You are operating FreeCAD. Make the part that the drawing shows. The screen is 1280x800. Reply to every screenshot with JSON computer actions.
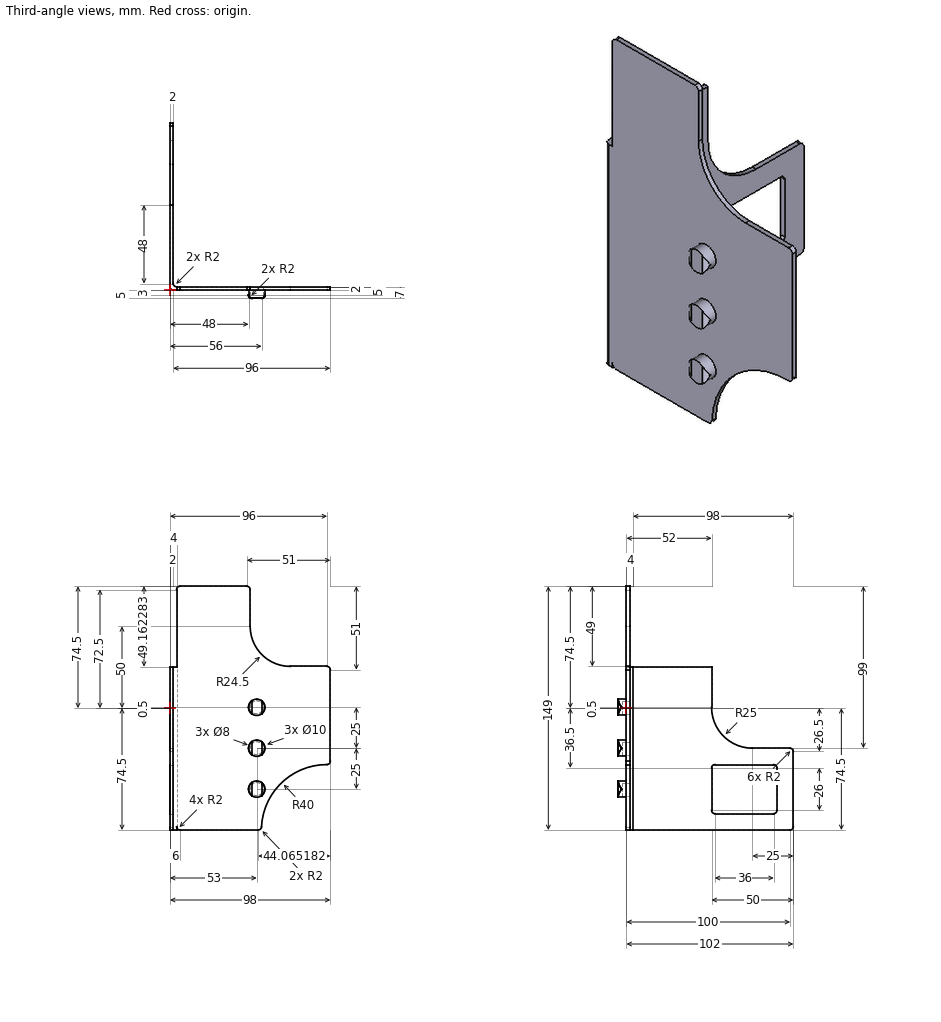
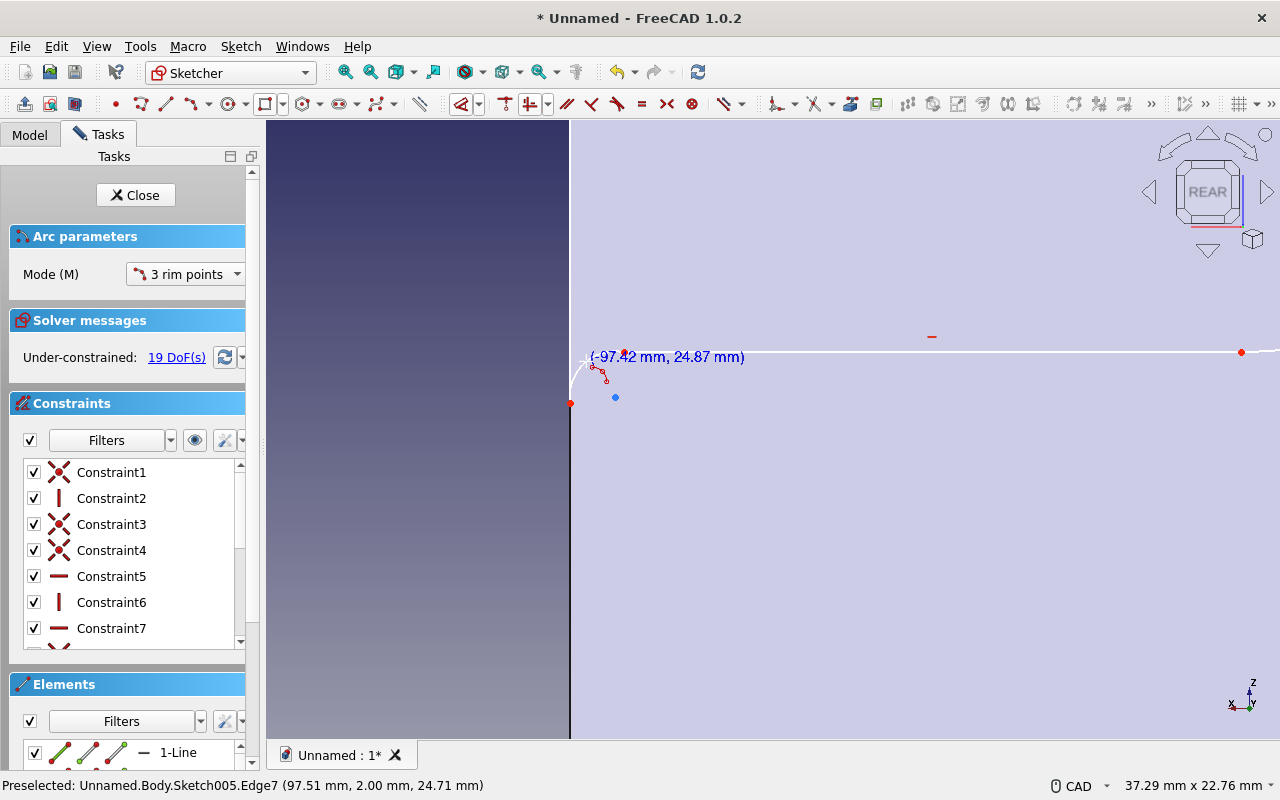
{"action": "left_click", "coordinate": [141, 104]}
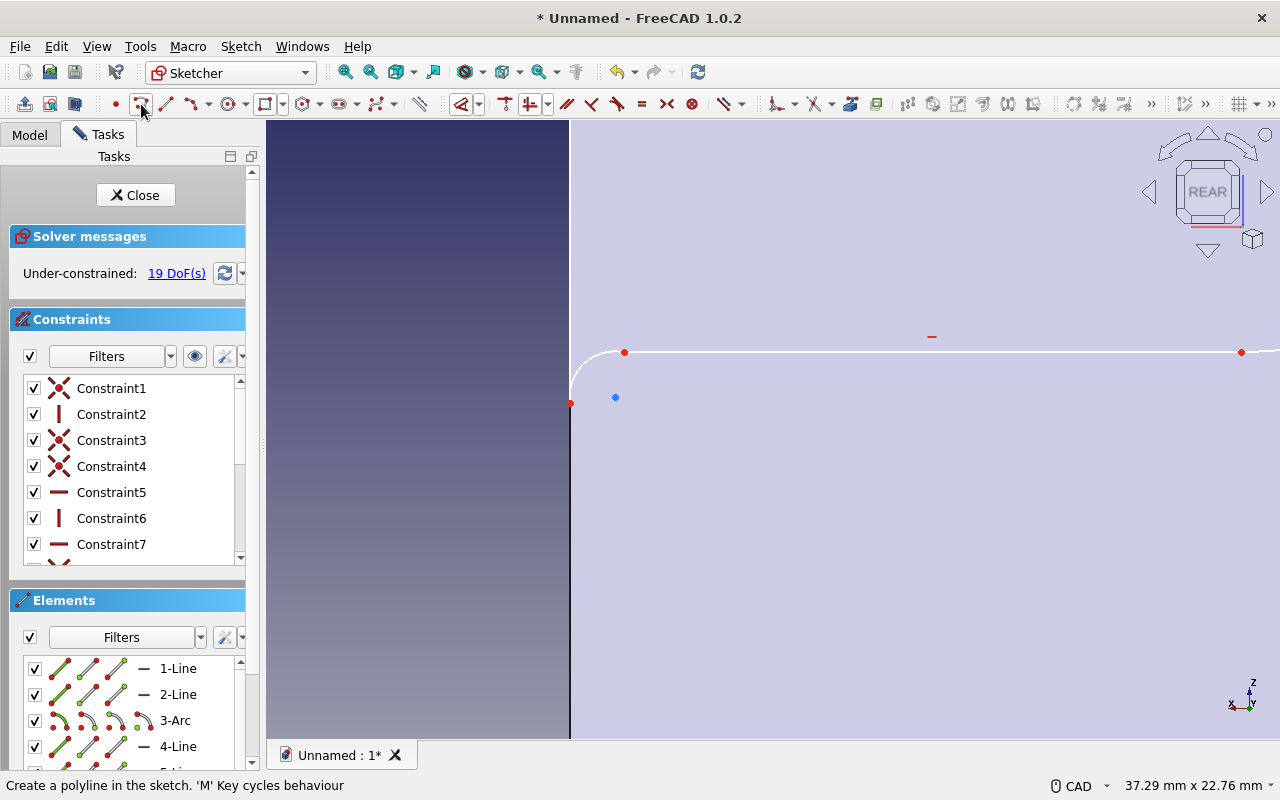
{"action": "scroll", "coordinate": [585, 369], "scroll_direction": "down", "scroll_amount": 12}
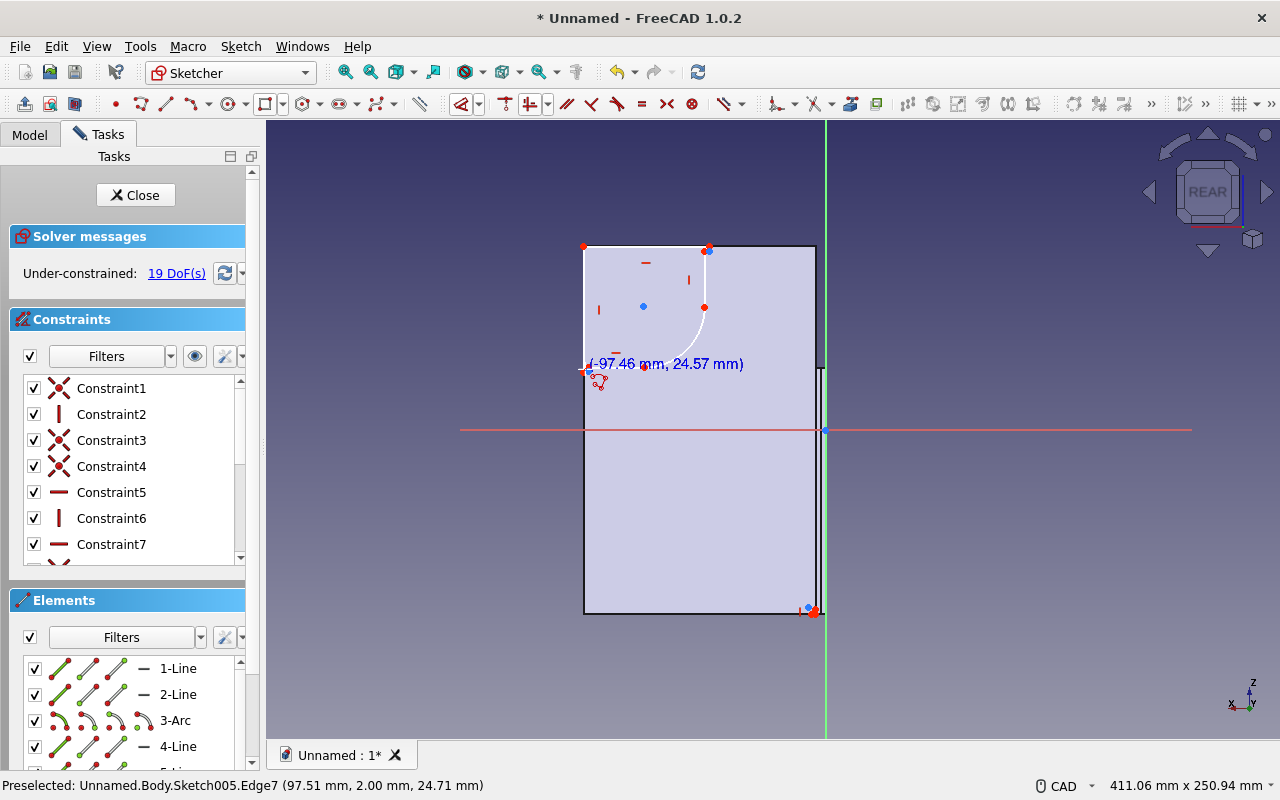
{"action": "scroll", "coordinate": [816, 251], "scroll_direction": "up", "scroll_amount": 3}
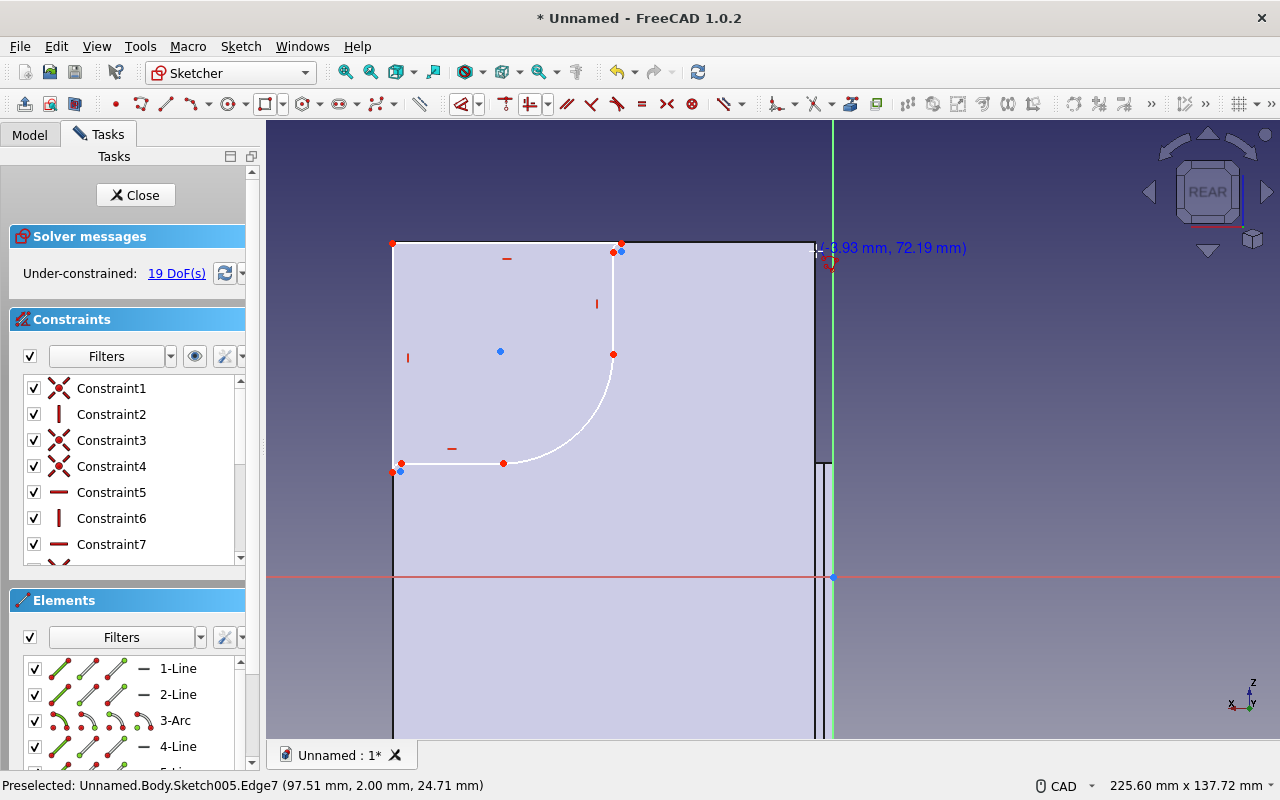
{"action": "left_click", "coordinate": [815, 251]}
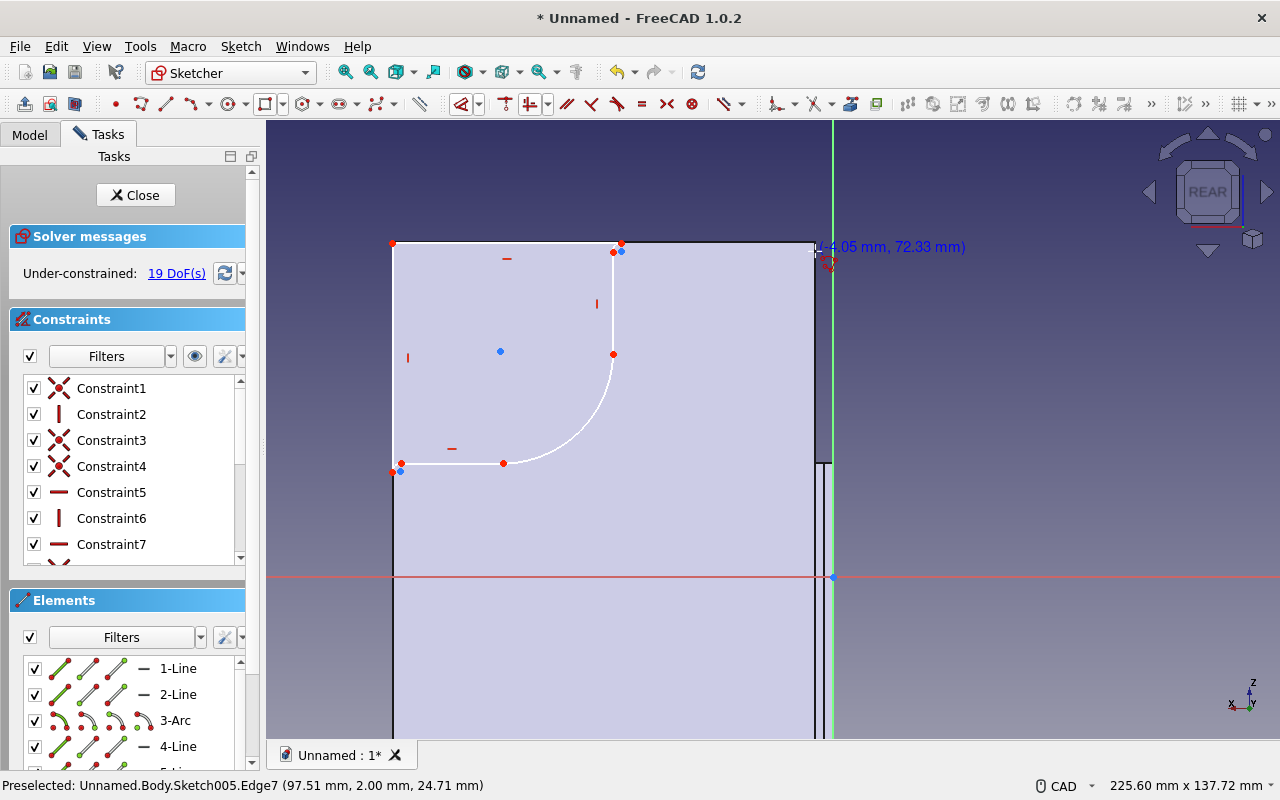
{"action": "scroll", "coordinate": [815, 242], "scroll_direction": "up", "scroll_amount": 3}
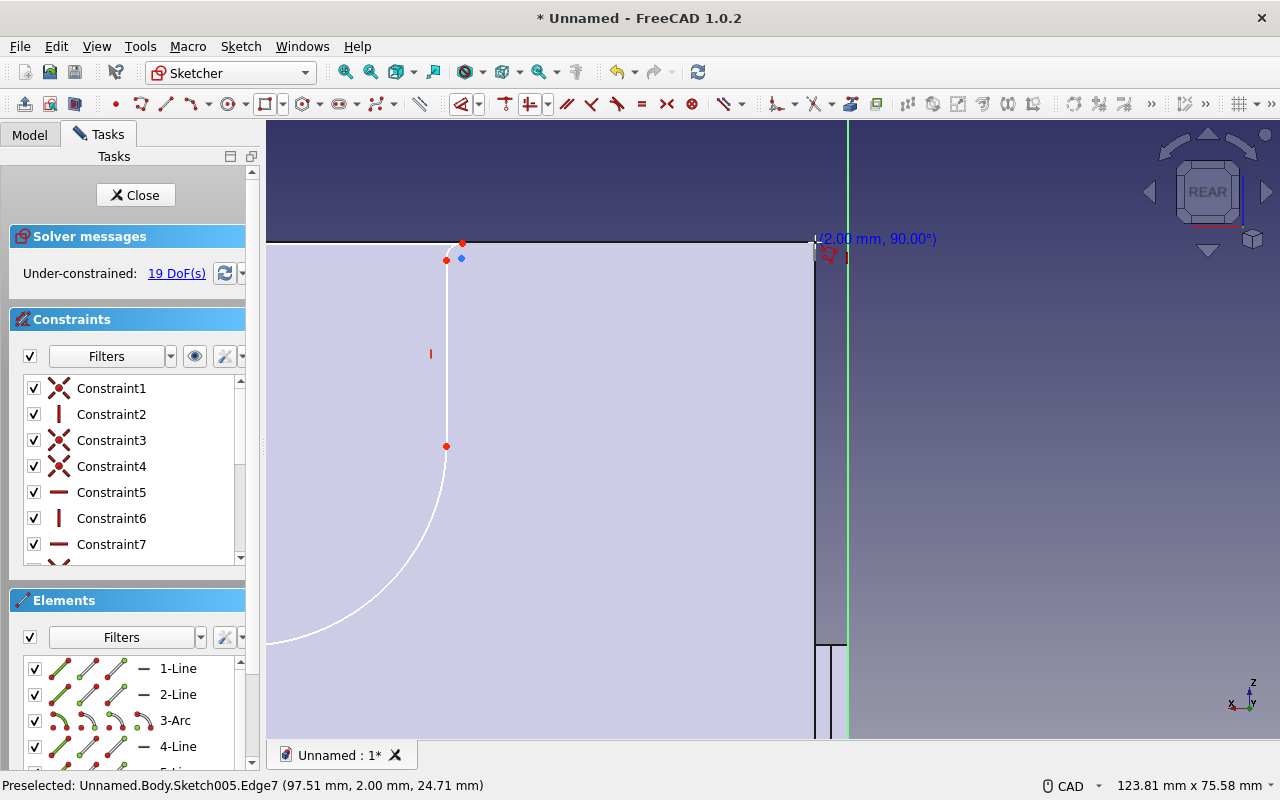
{"action": "left_click", "coordinate": [815, 242]}
{"action": "left_click", "coordinate": [799, 242]}
{"action": "right_click", "coordinate": [799, 242]}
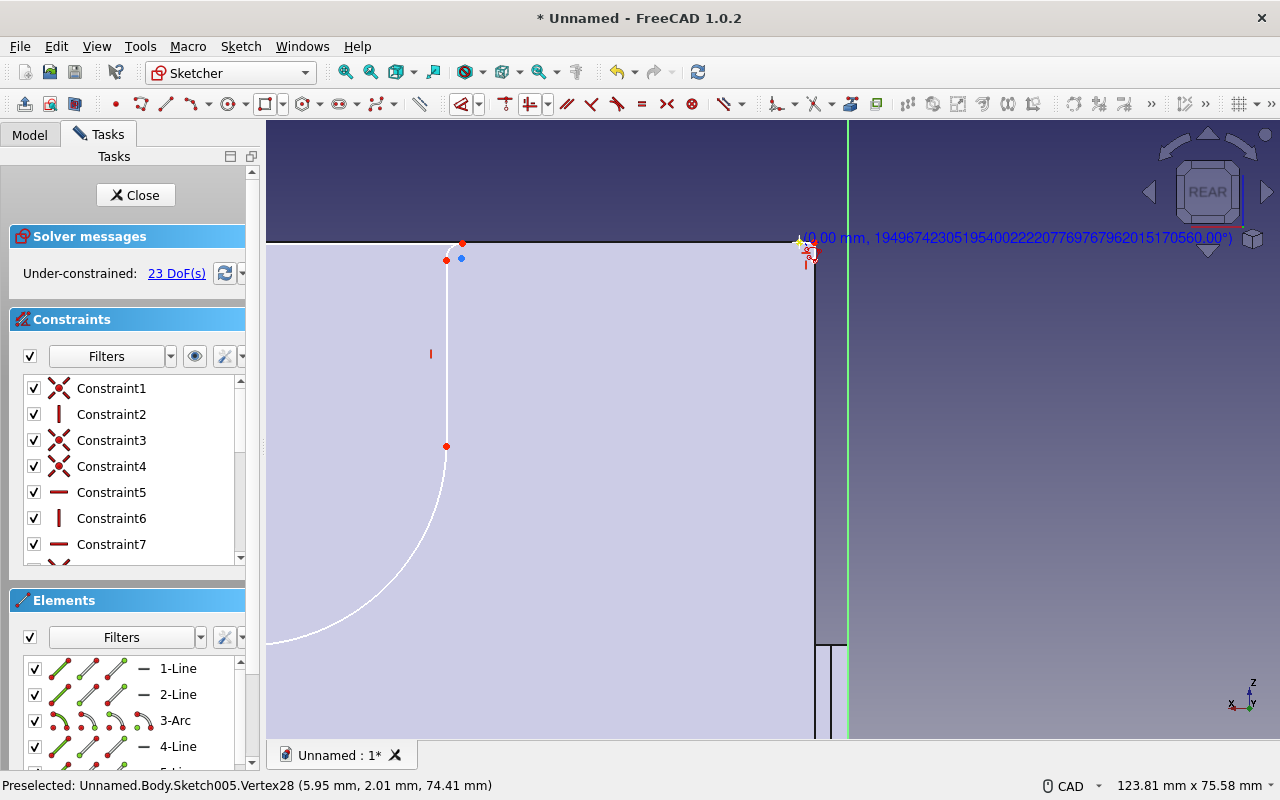
{"action": "key", "text": "g 3 a"}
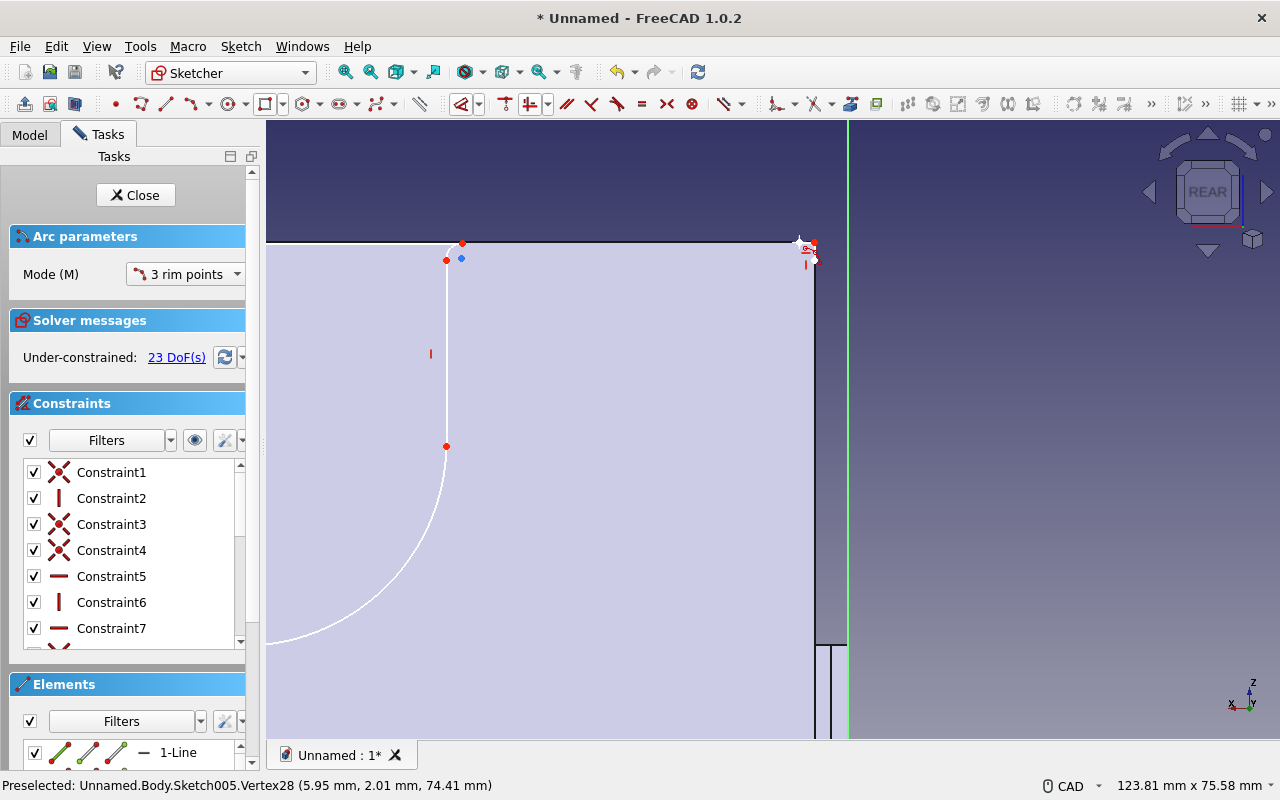
{"action": "scroll", "coordinate": [799, 242], "scroll_direction": "up", "scroll_amount": 4}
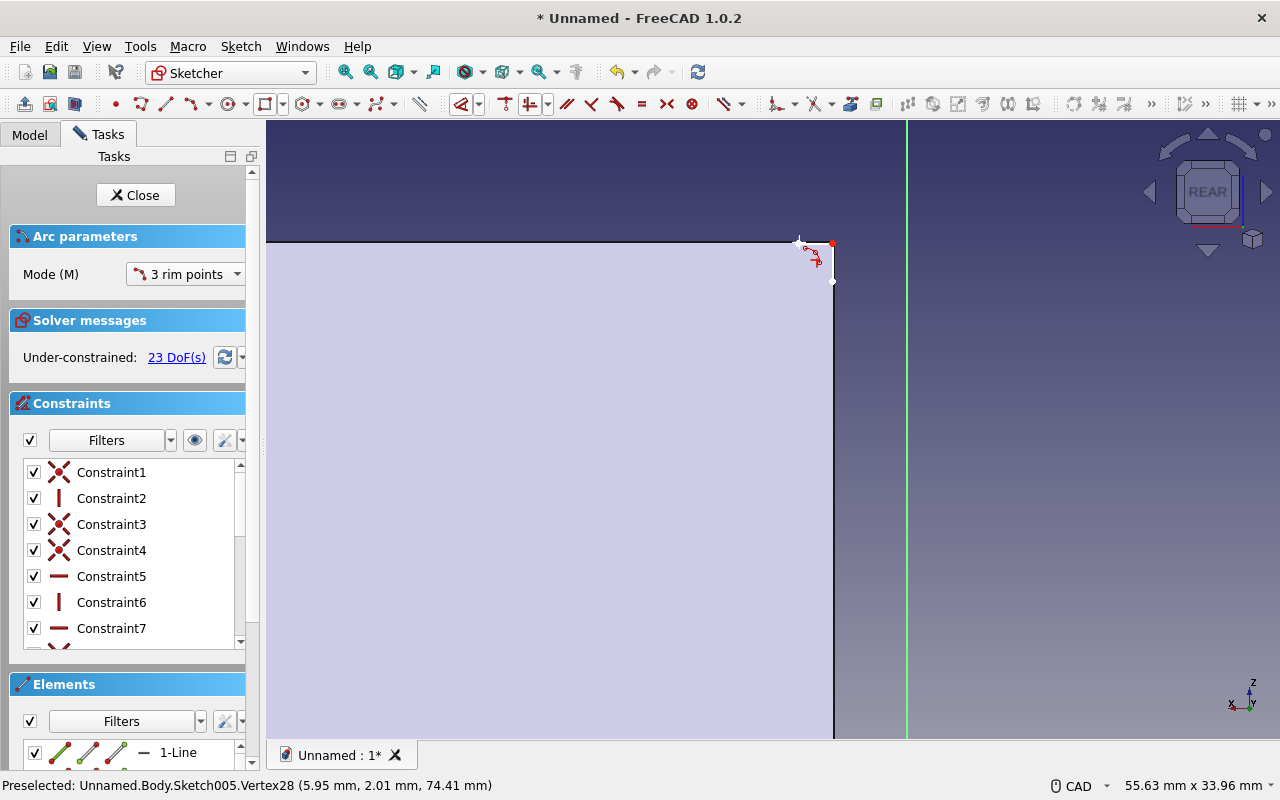
{"action": "left_click", "coordinate": [798, 244]}
{"action": "left_click", "coordinate": [833, 282]}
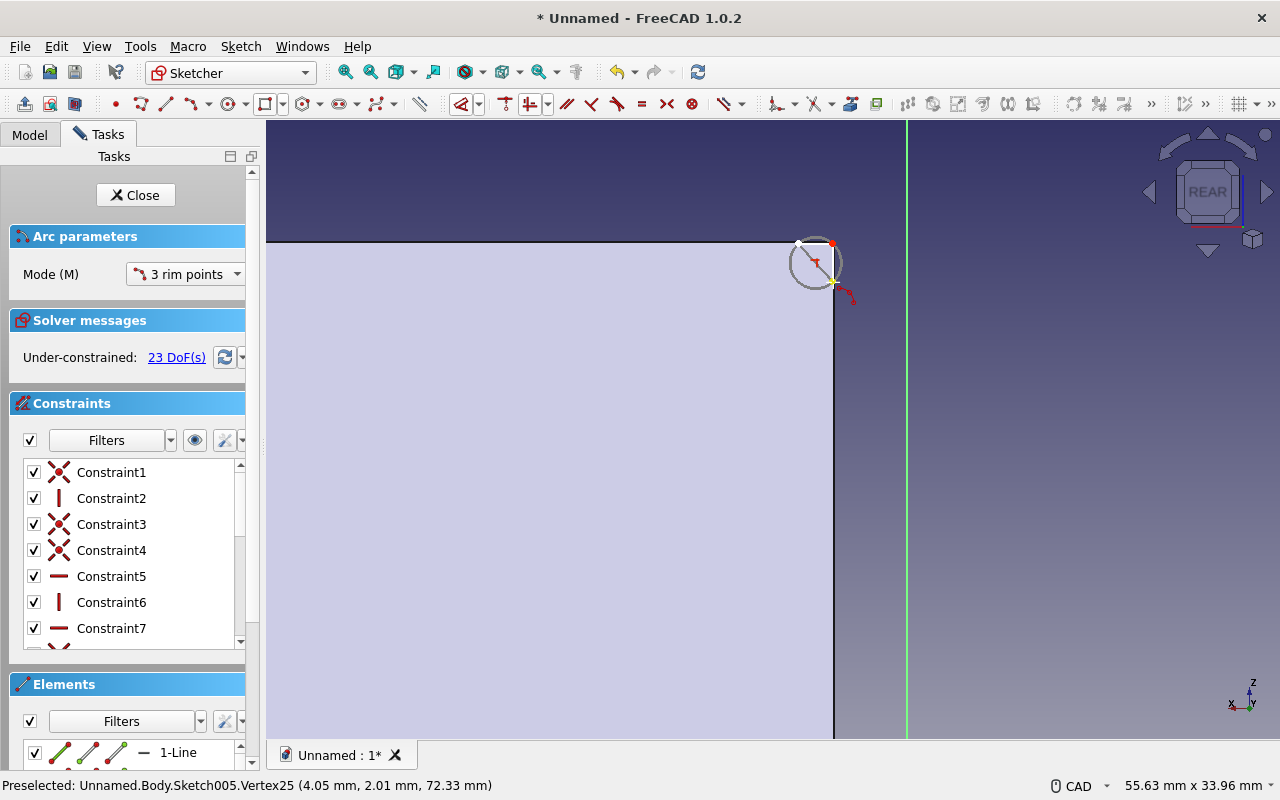
{"action": "scroll", "coordinate": [823, 253], "scroll_direction": "up", "scroll_amount": 2}